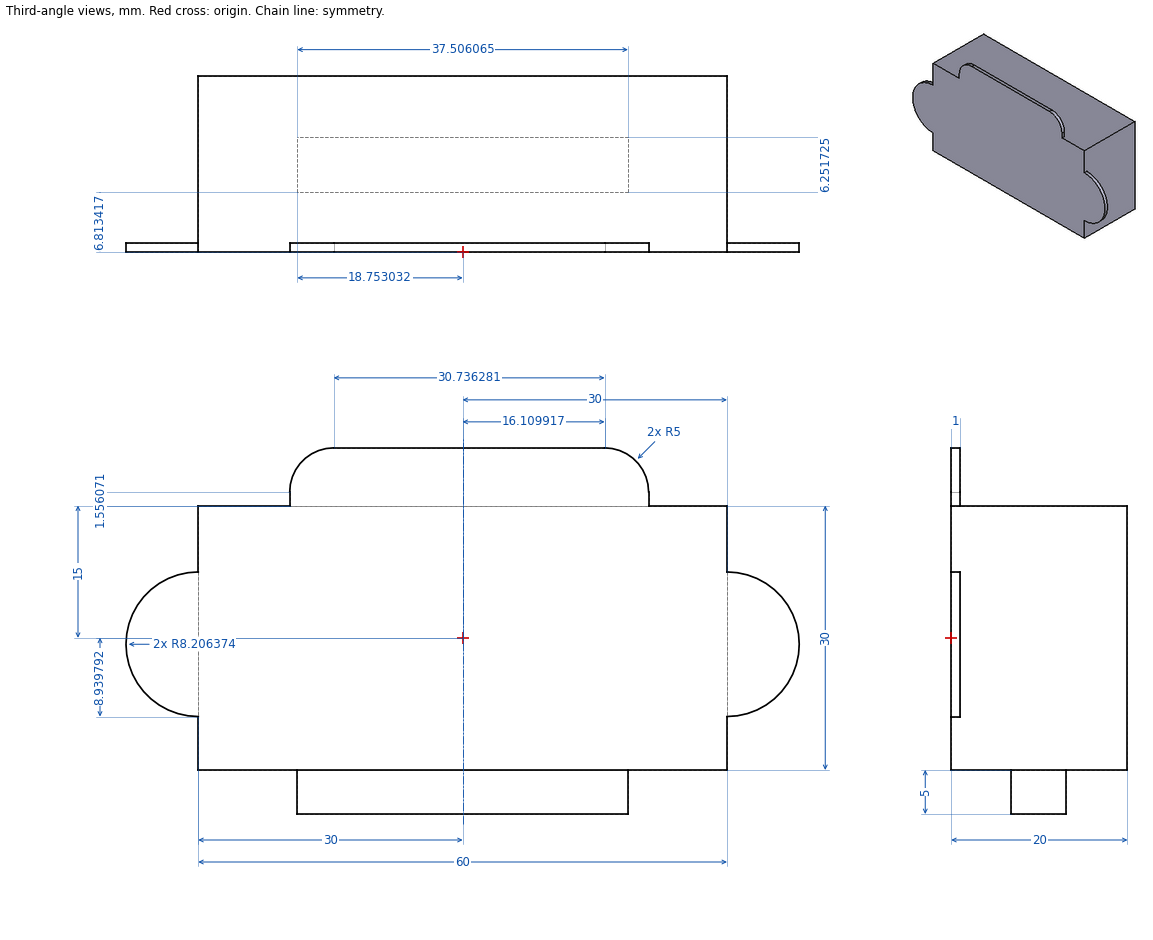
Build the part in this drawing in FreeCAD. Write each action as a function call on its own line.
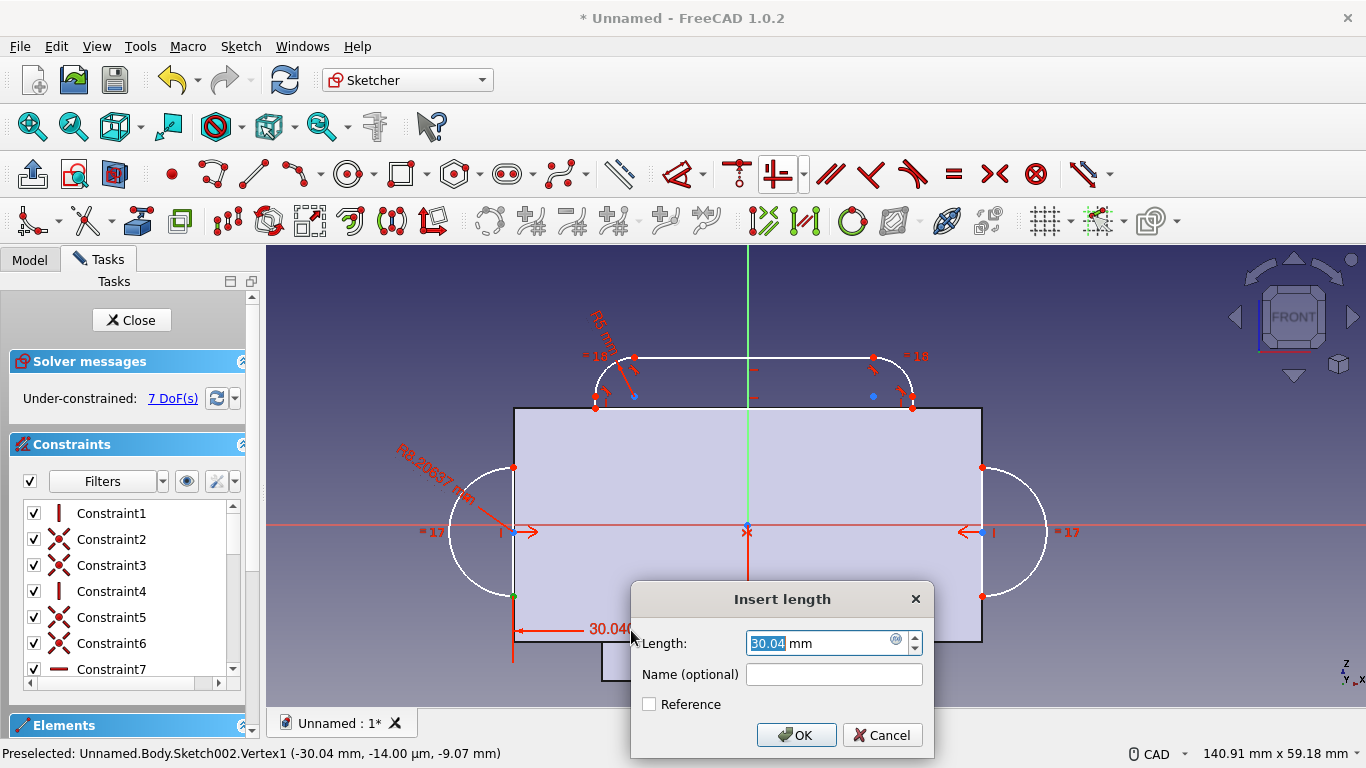
text(30)
key(Return)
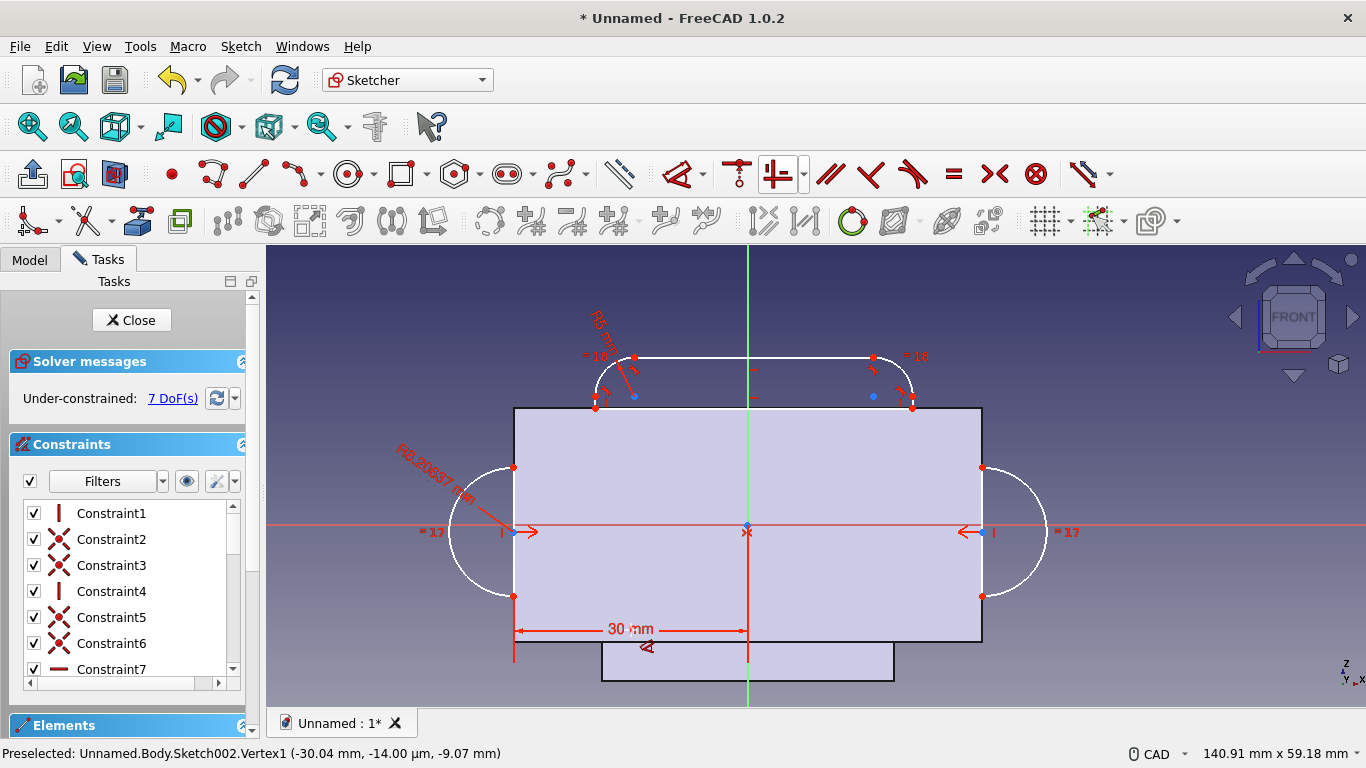
click(982, 468)
click(865, 559)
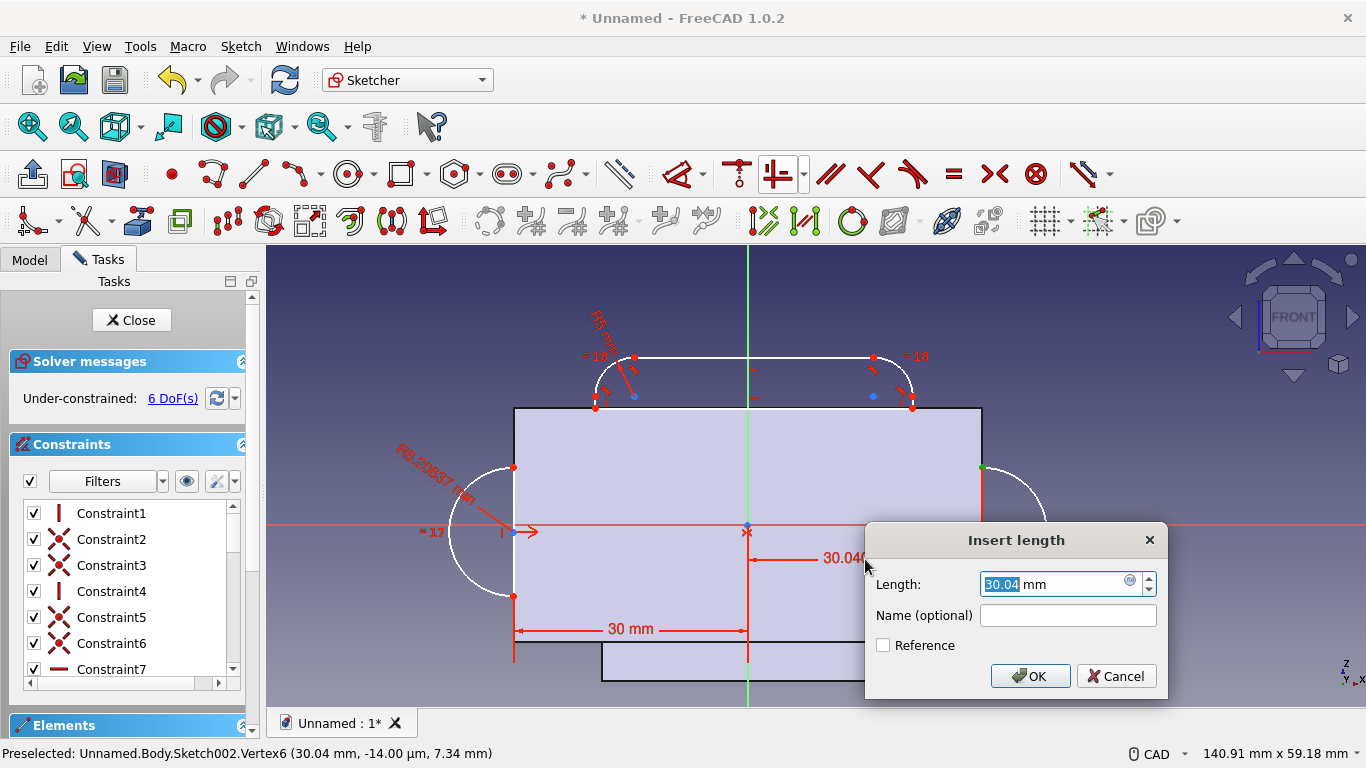
text(30)
key(Return)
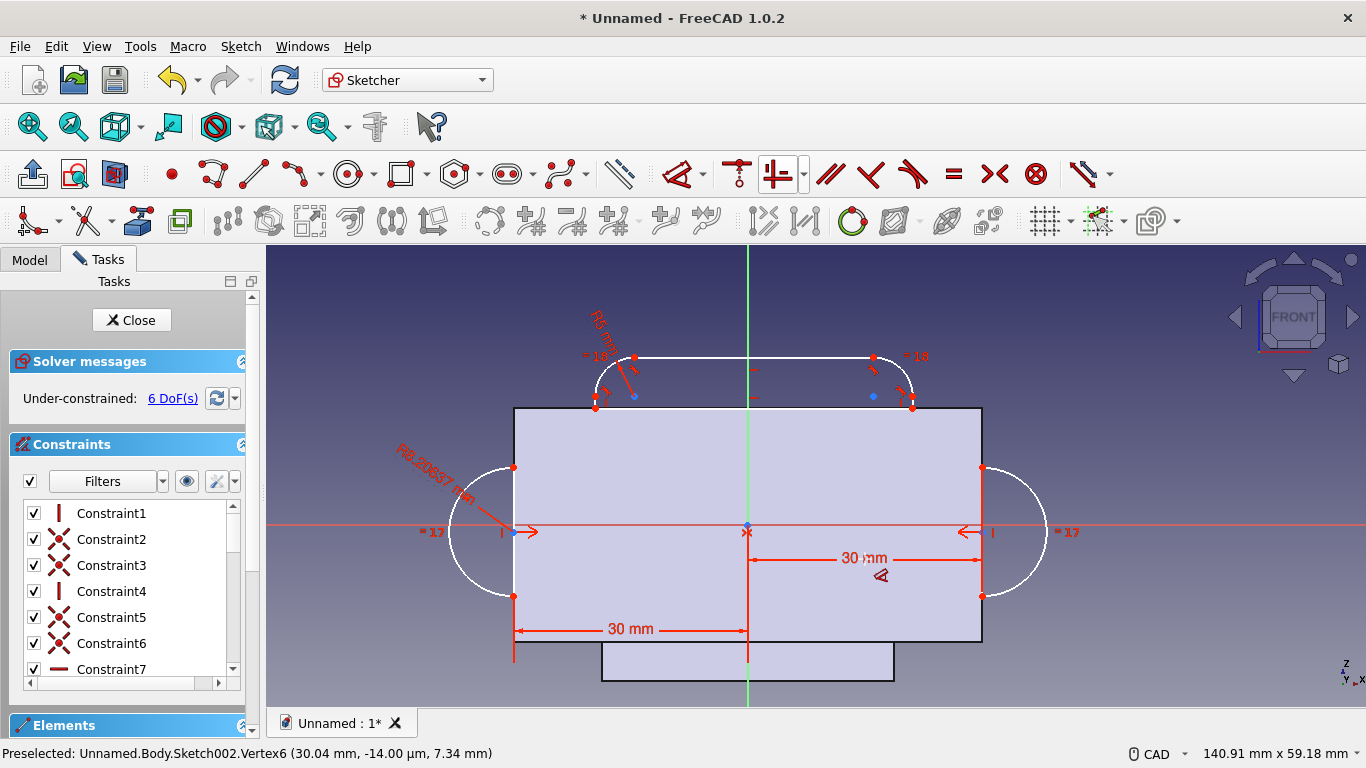
click(595, 409)
click(561, 467)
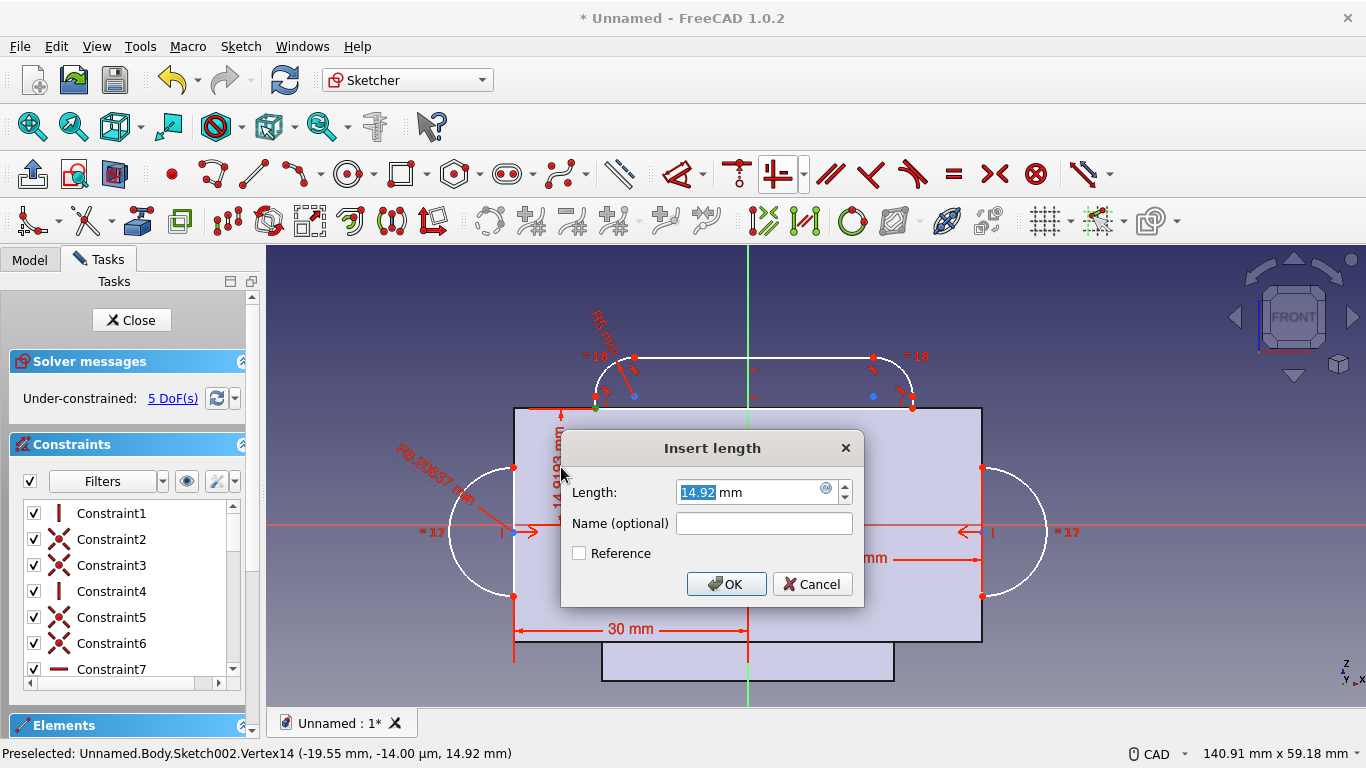
text(15)
key(Return)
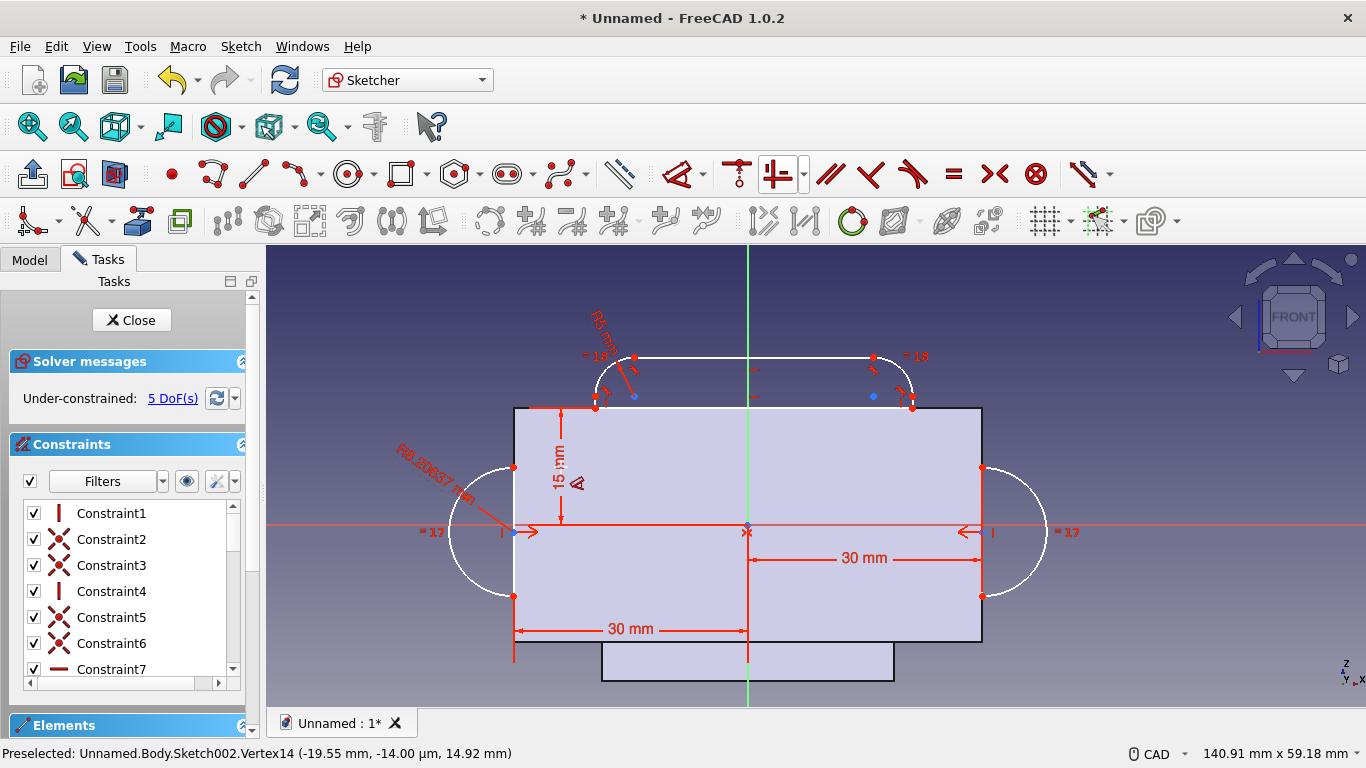
click(513, 532)
click(631, 566)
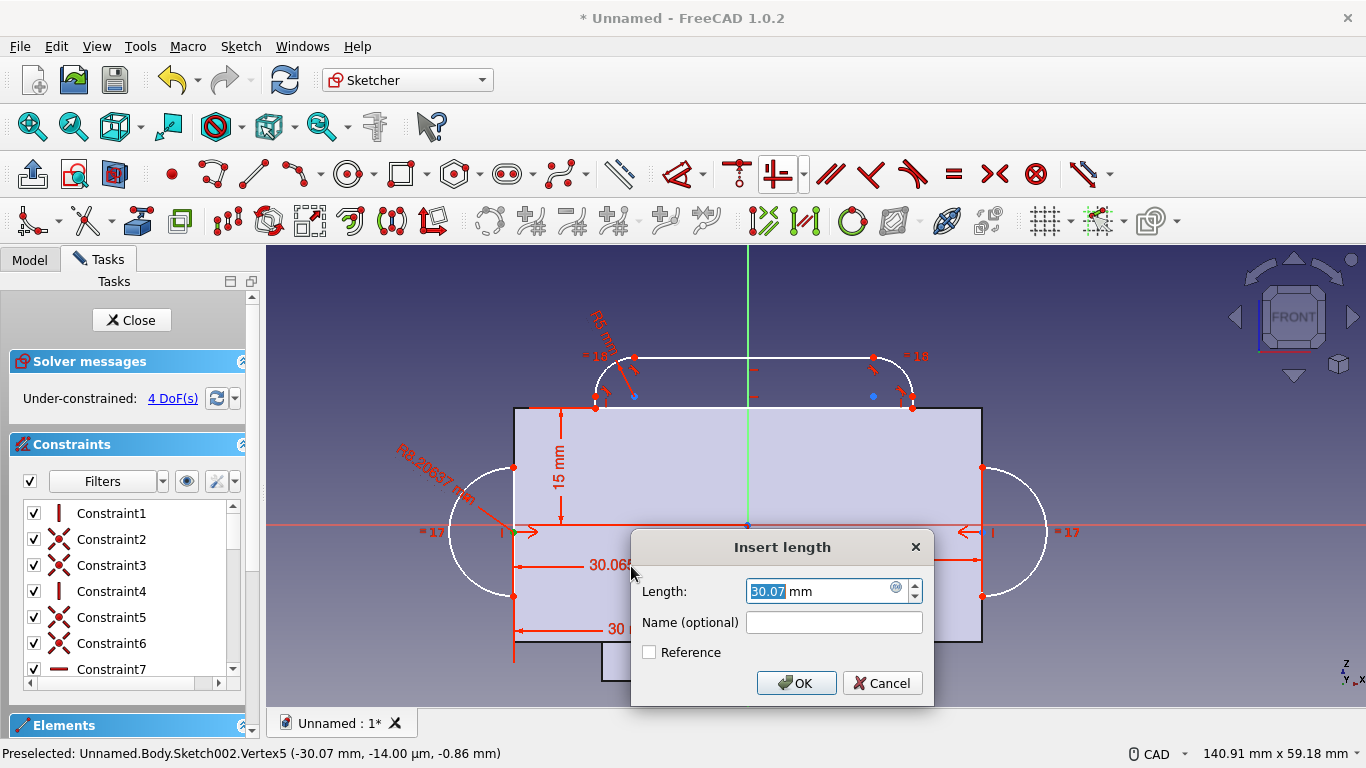
text(30)
key(Return)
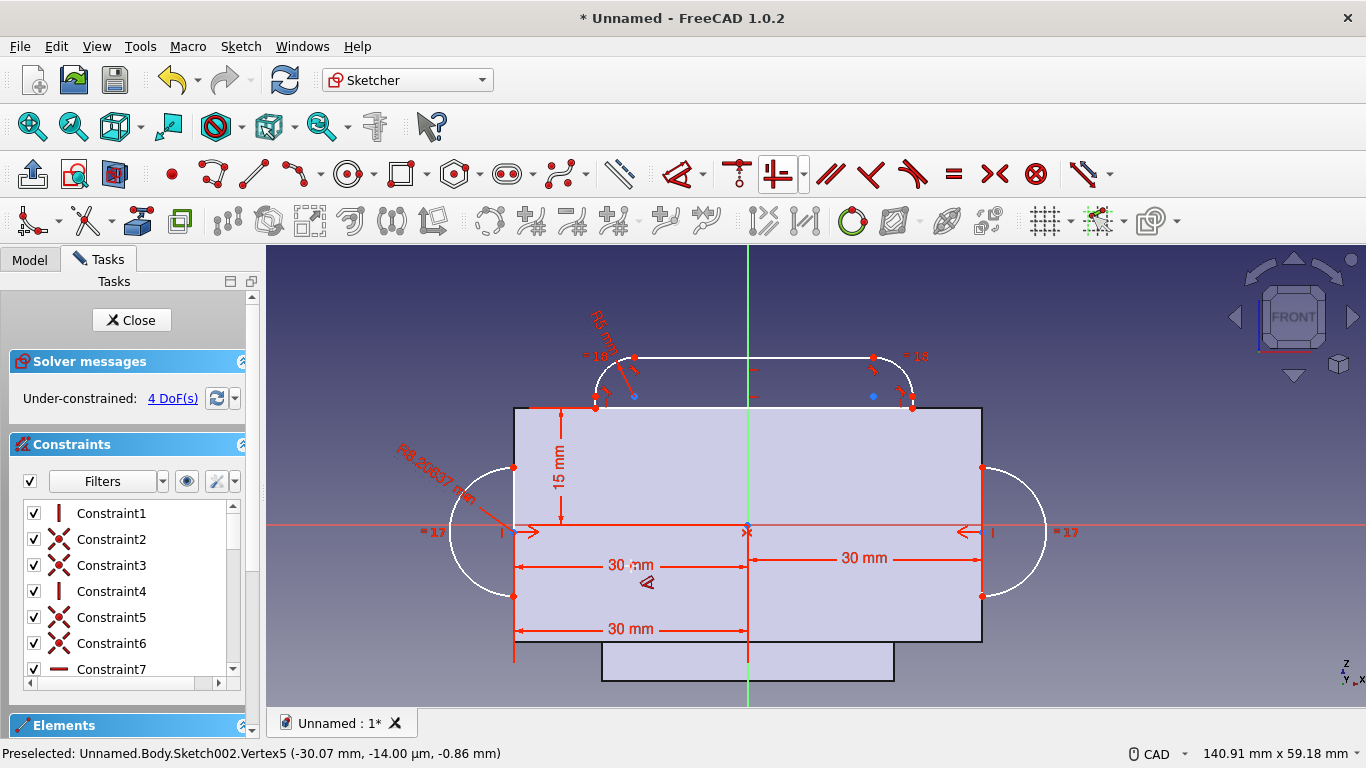
scroll(595, 402, up, 6)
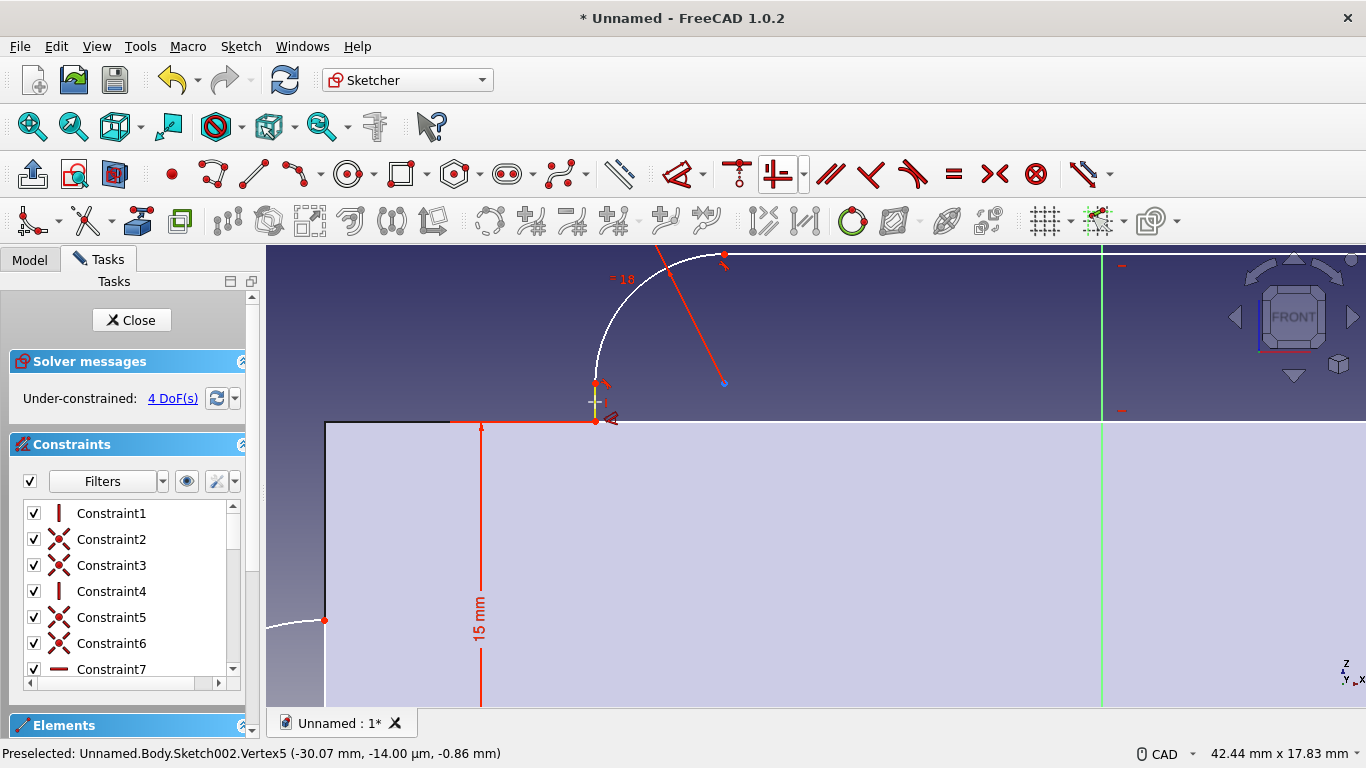
click(595, 403)
click(561, 403)